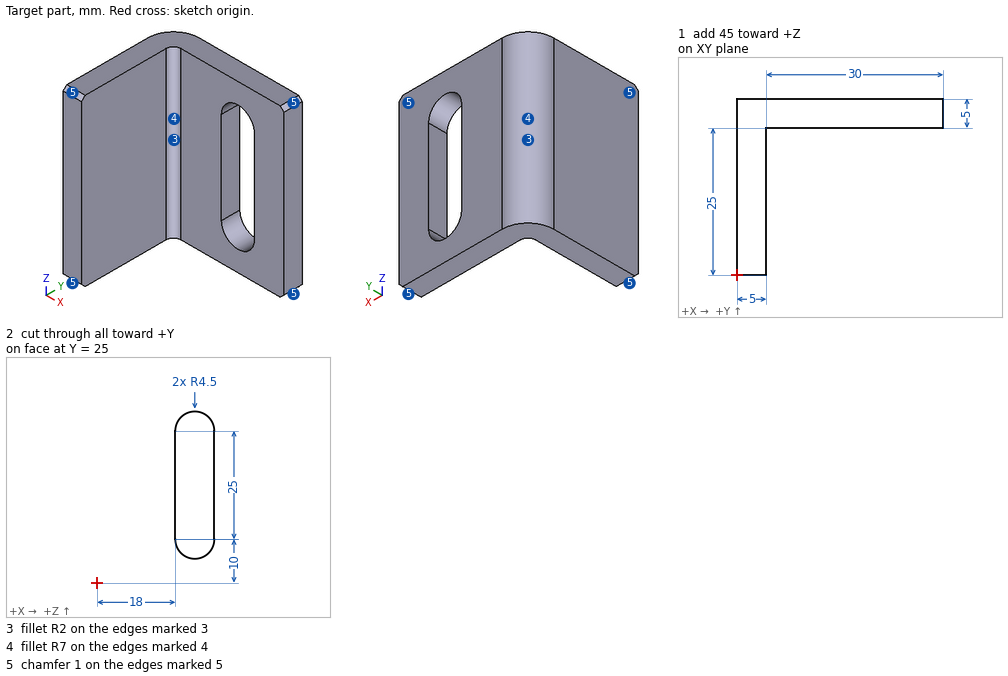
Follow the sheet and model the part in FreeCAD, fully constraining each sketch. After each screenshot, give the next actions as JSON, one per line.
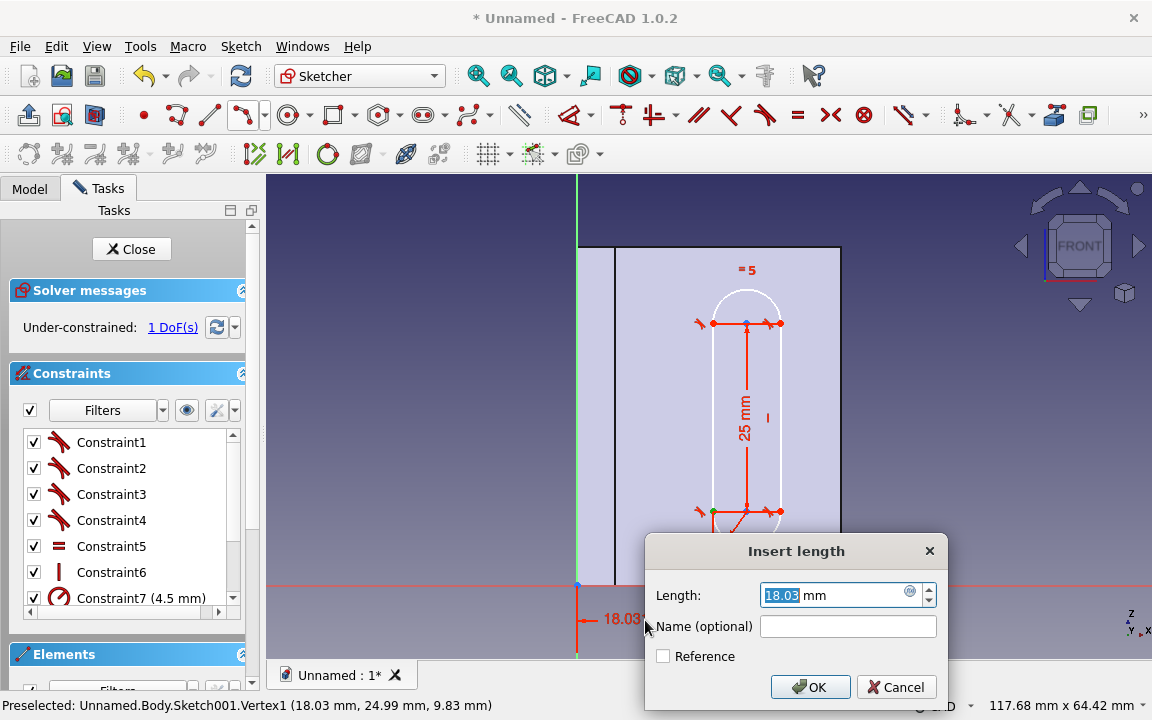
{"action": "type", "text": "18"}
{"action": "key", "text": "Return"}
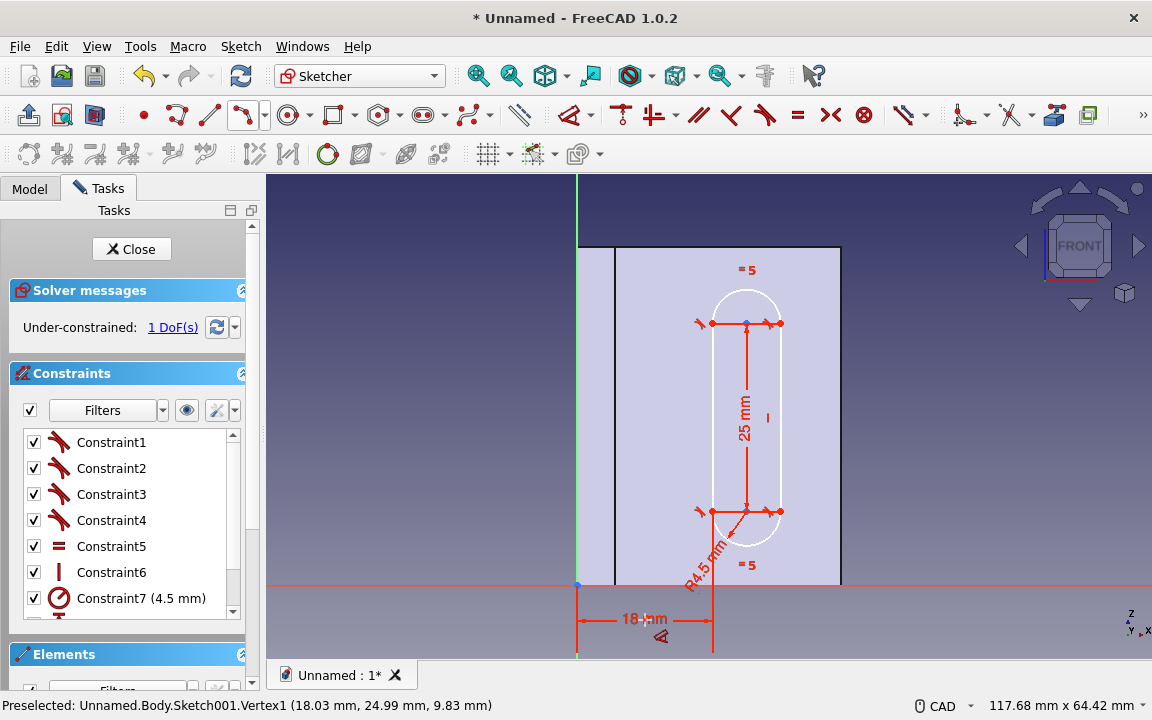
{"action": "left_click", "coordinate": [713, 512]}
{"action": "left_click", "coordinate": [543, 549]}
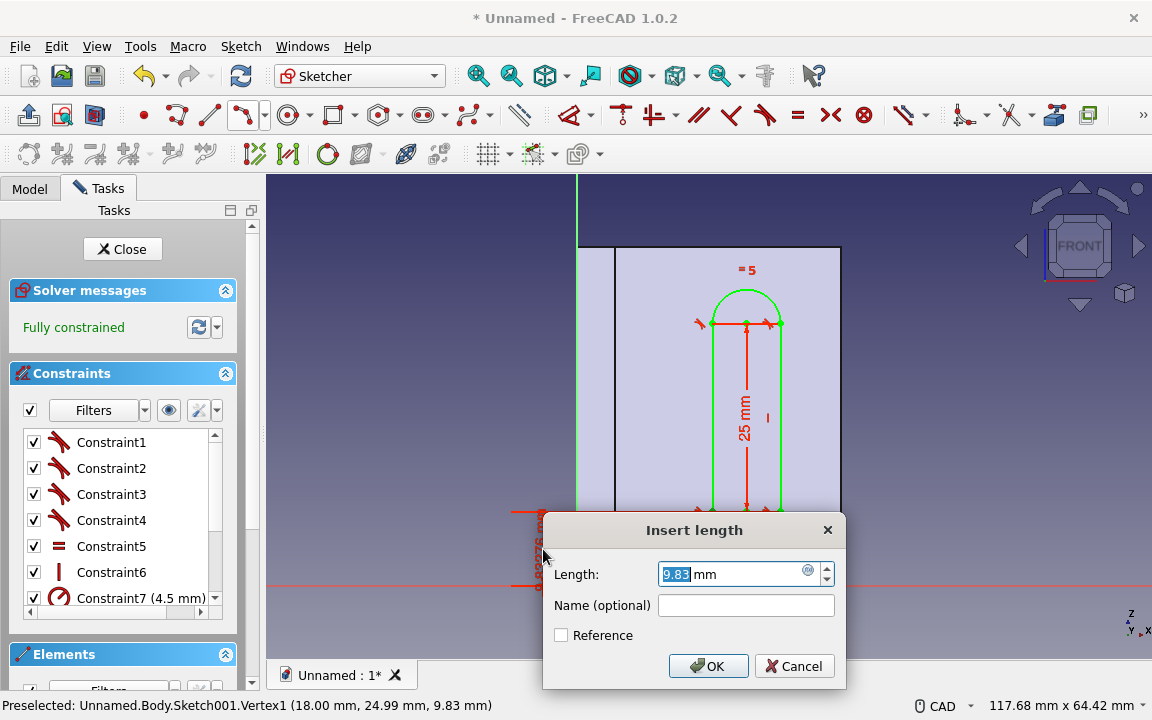
{"action": "type", "text": "10"}
{"action": "key", "text": "Return"}
{"action": "key", "text": "Escape"}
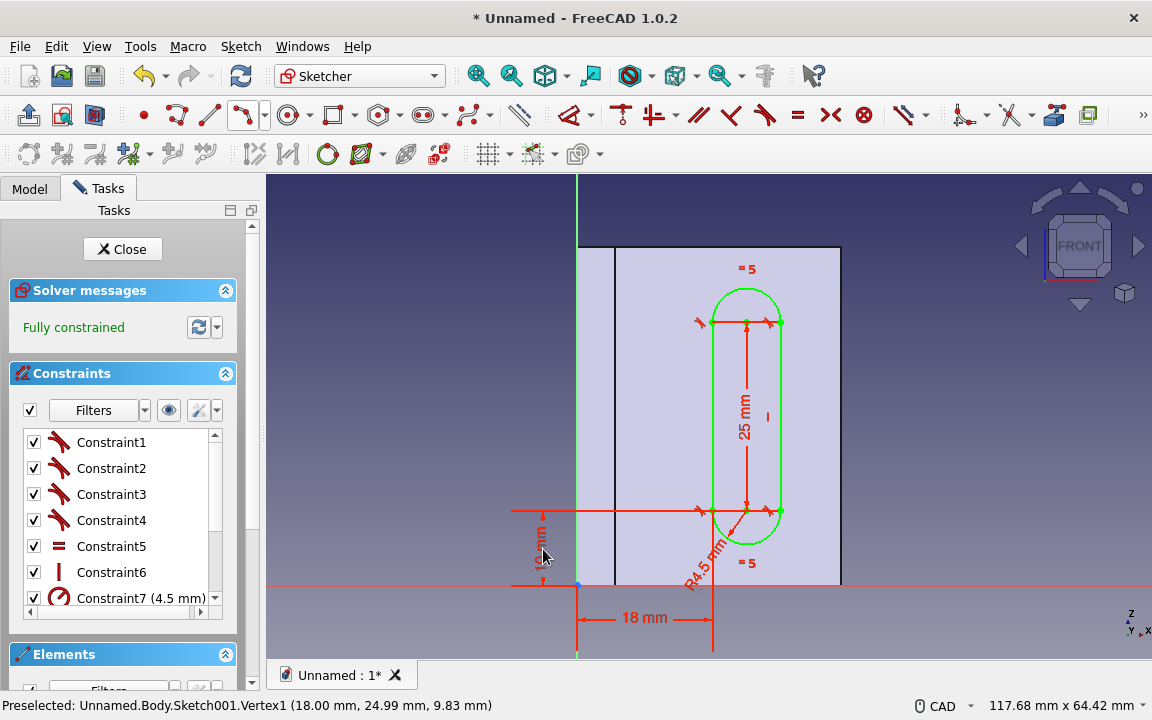
{"action": "left_click", "coordinate": [123, 249]}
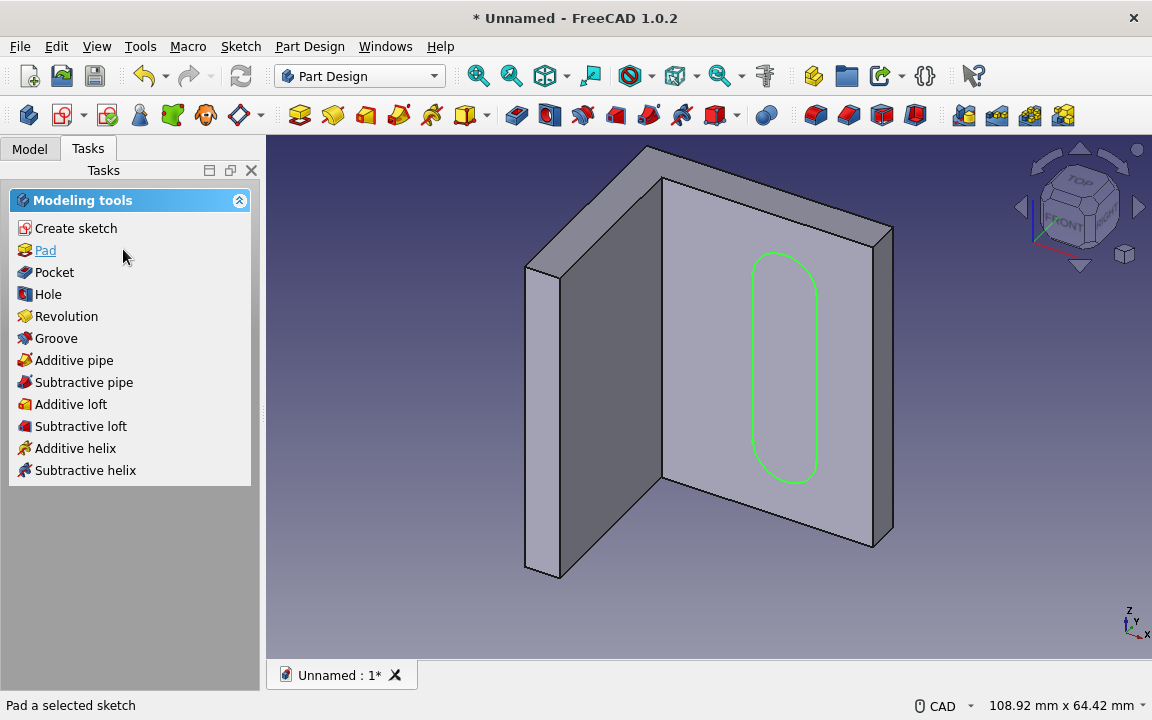
{"action": "left_click", "coordinate": [517, 116]}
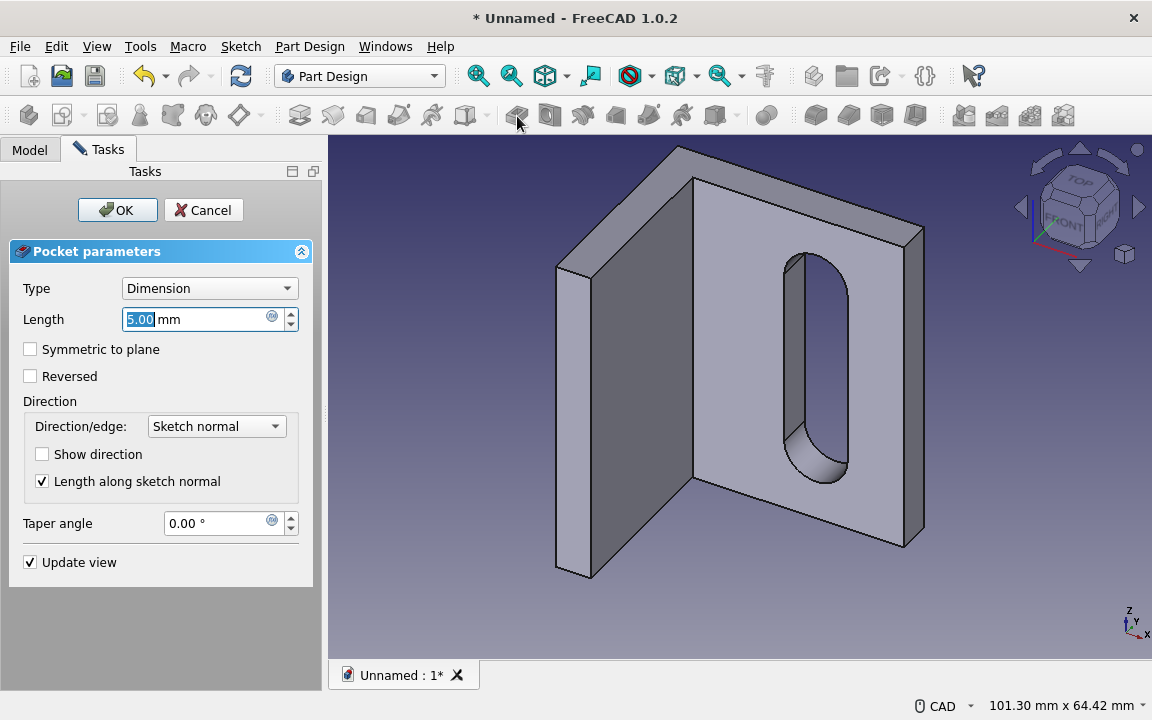
{"action": "left_click", "coordinate": [210, 288]}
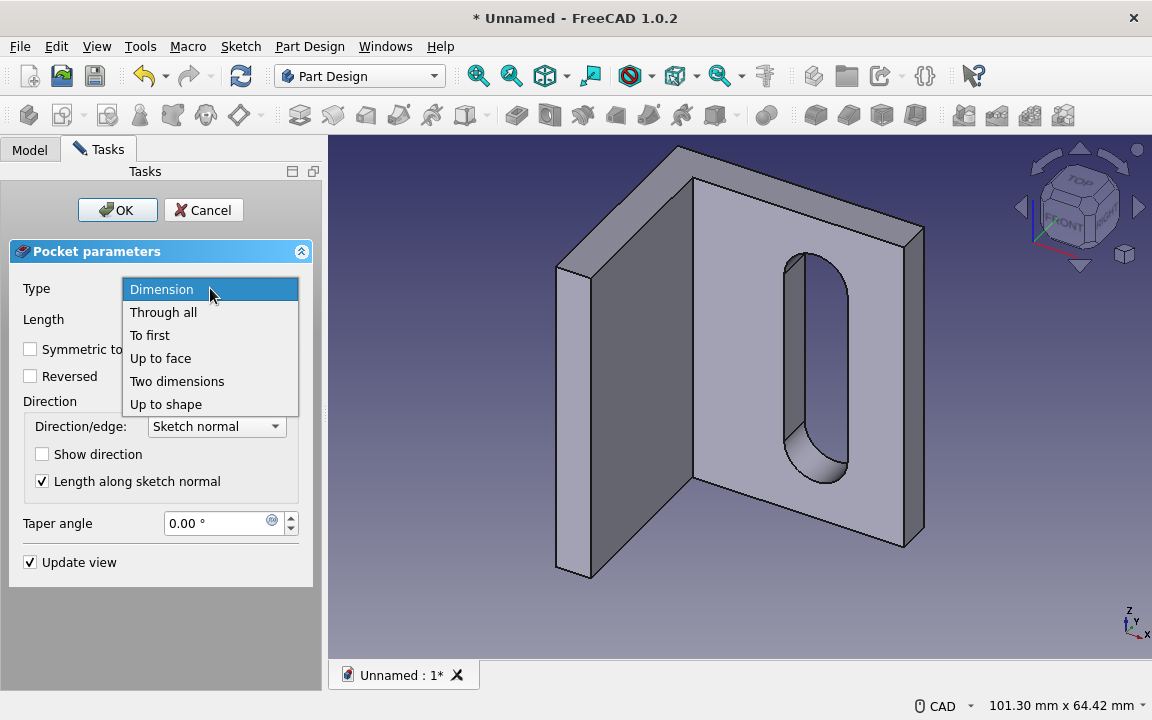
{"action": "left_click", "coordinate": [208, 312]}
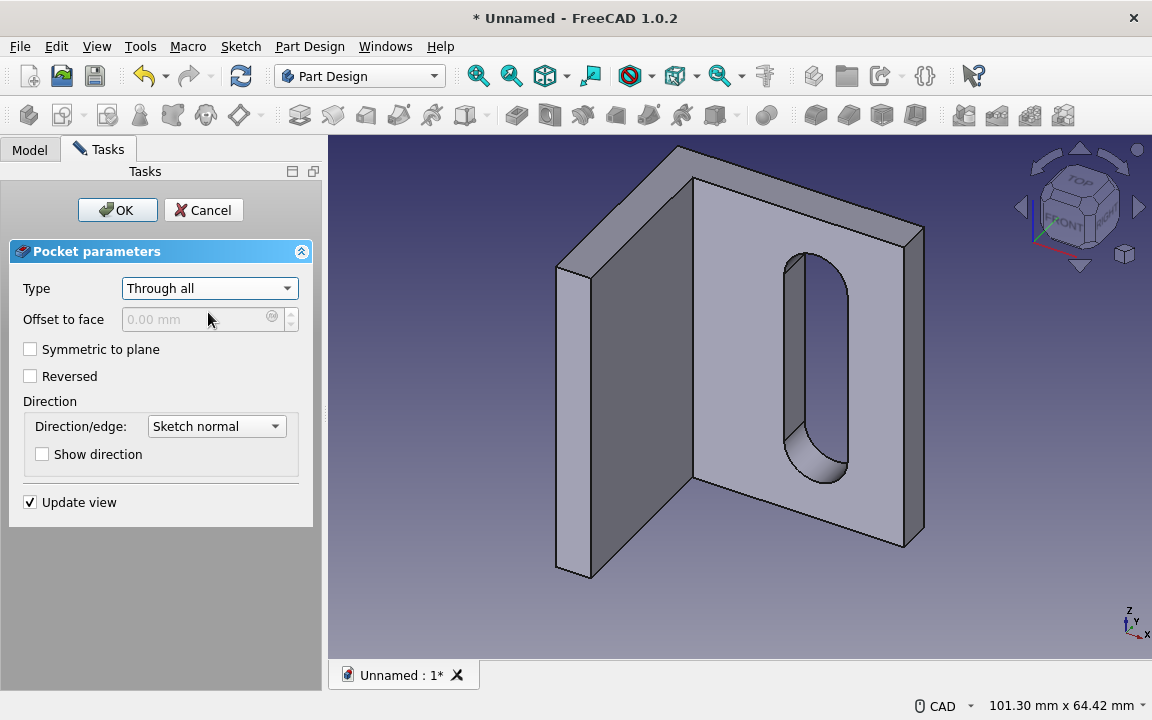
{"action": "left_click", "coordinate": [118, 210]}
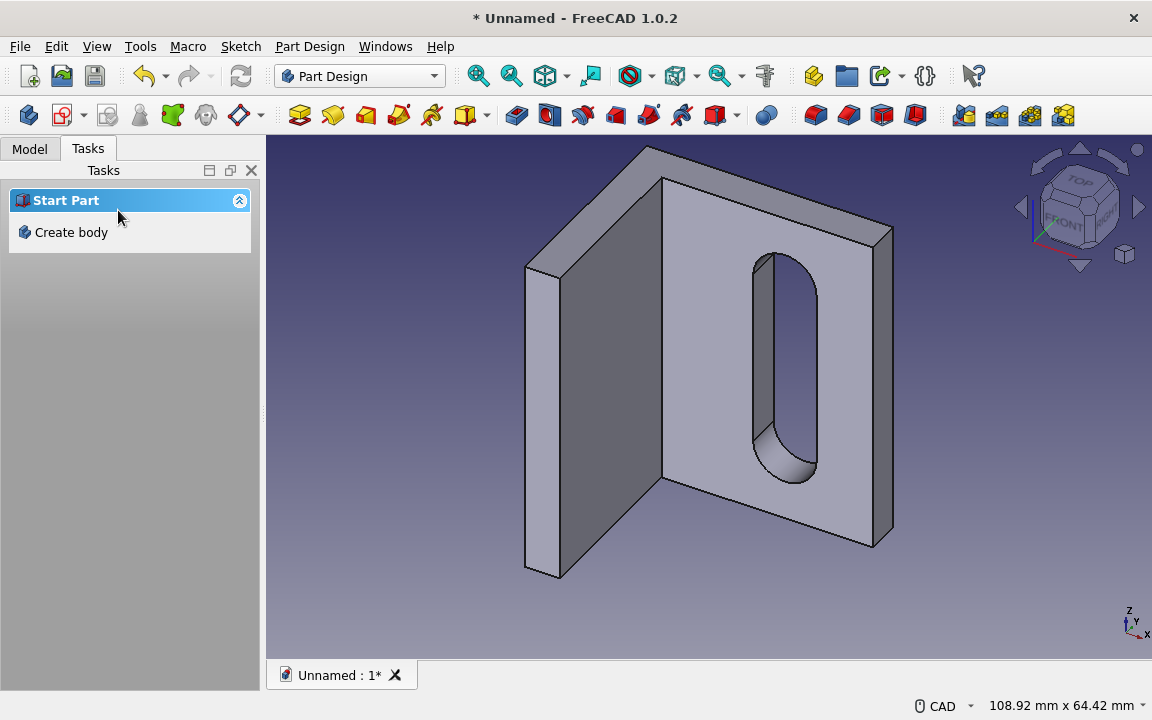
{"action": "key", "text": "0"}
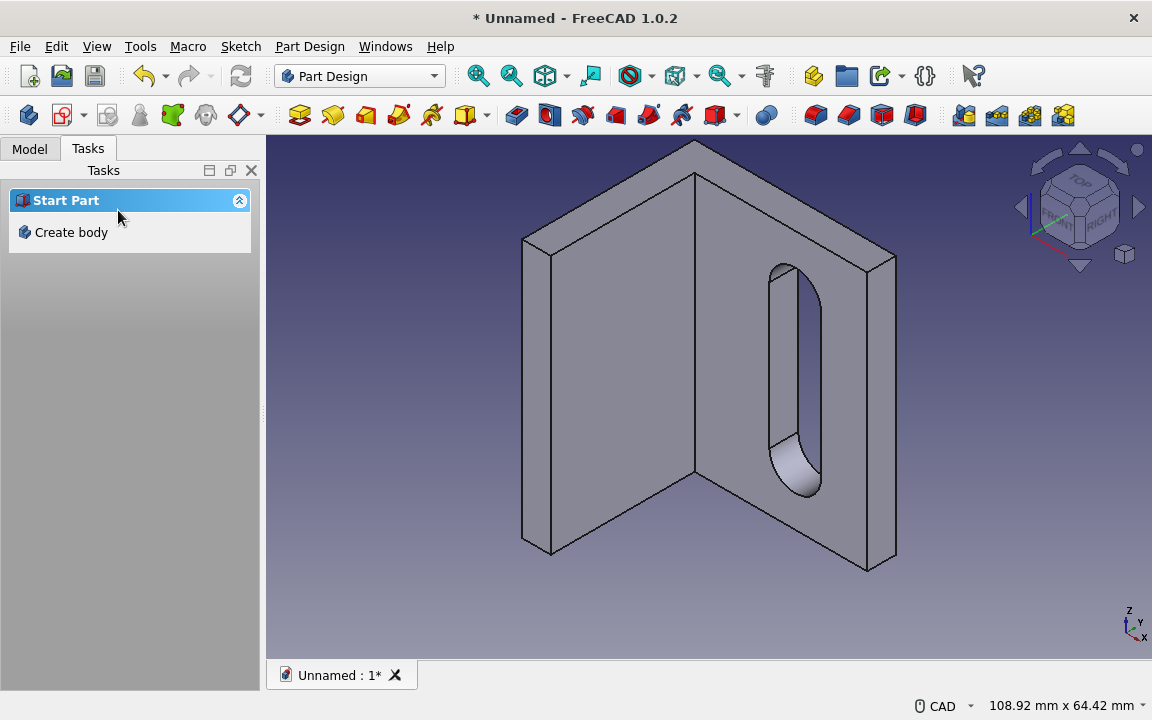
{"action": "key", "text": "2"}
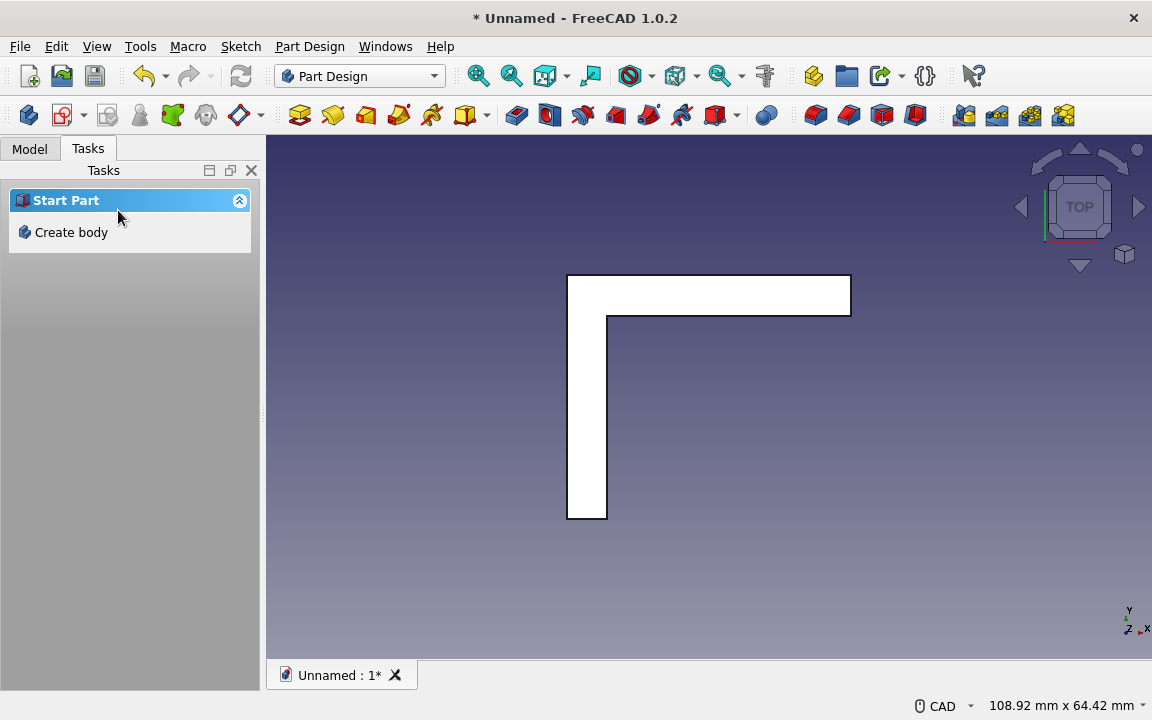
{"action": "key", "text": "1"}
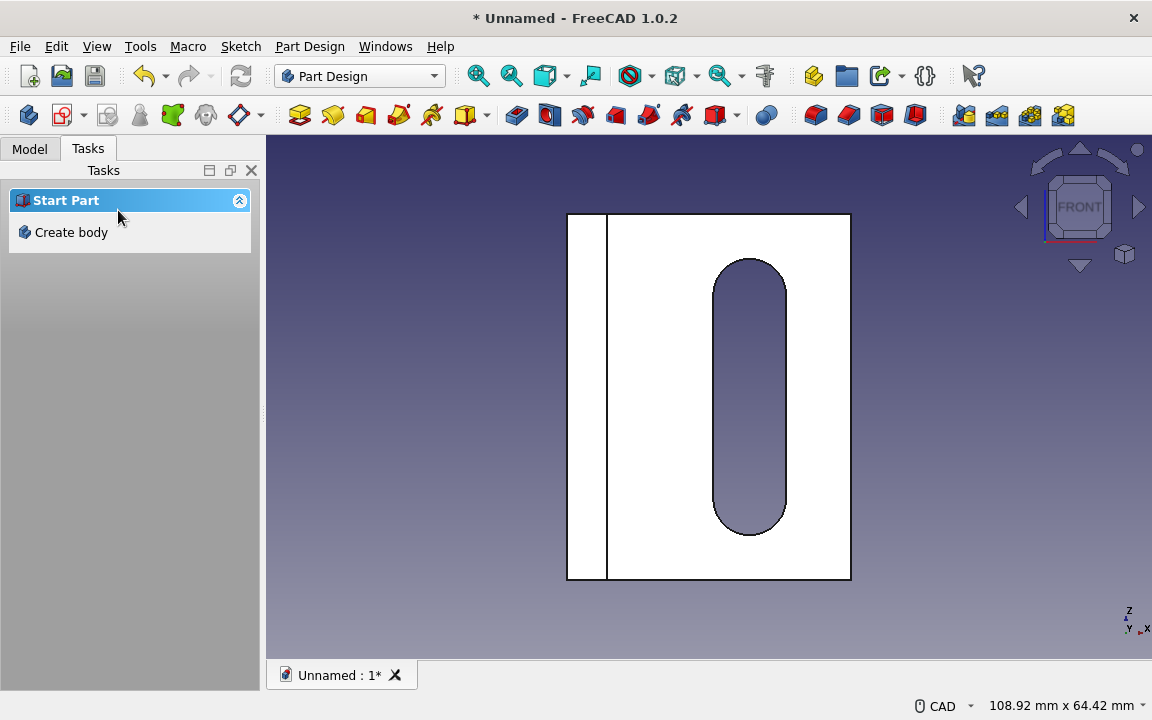
{"action": "key", "text": "3"}